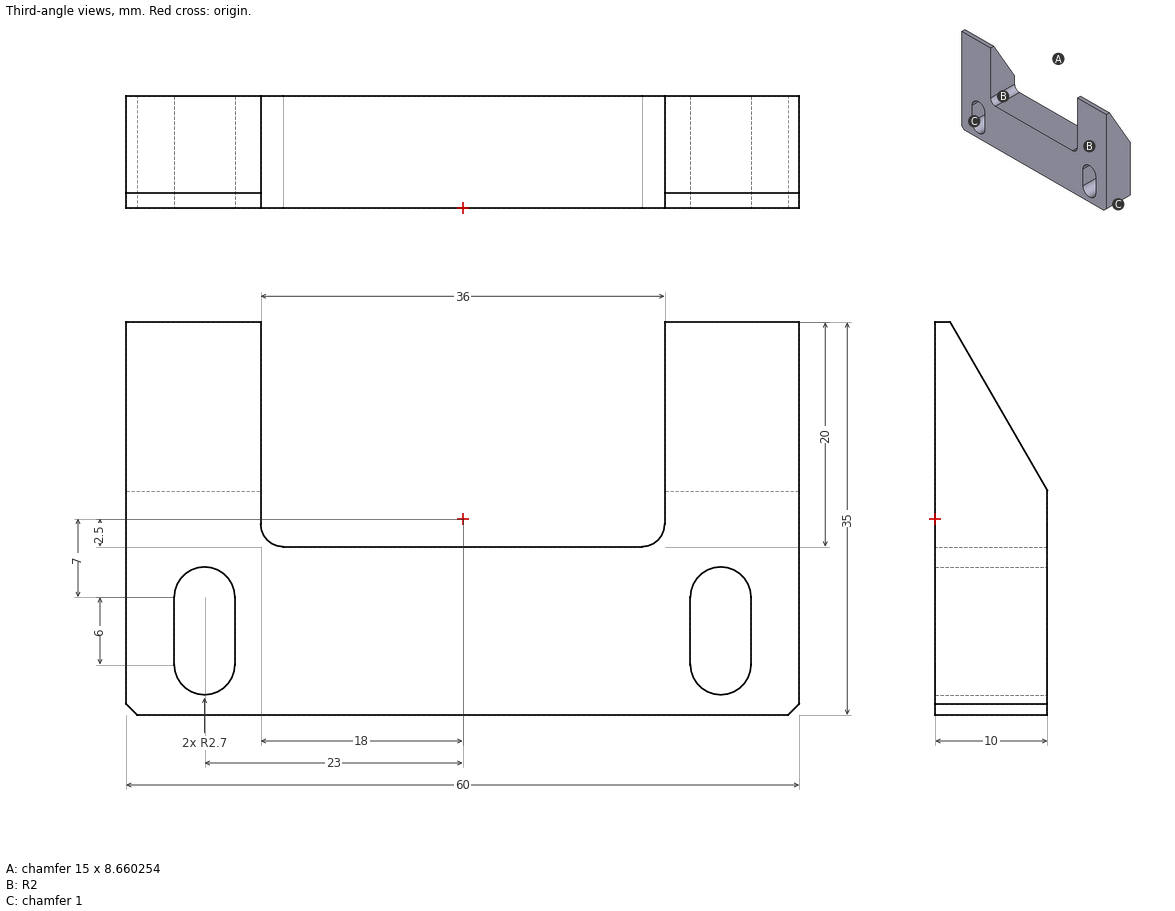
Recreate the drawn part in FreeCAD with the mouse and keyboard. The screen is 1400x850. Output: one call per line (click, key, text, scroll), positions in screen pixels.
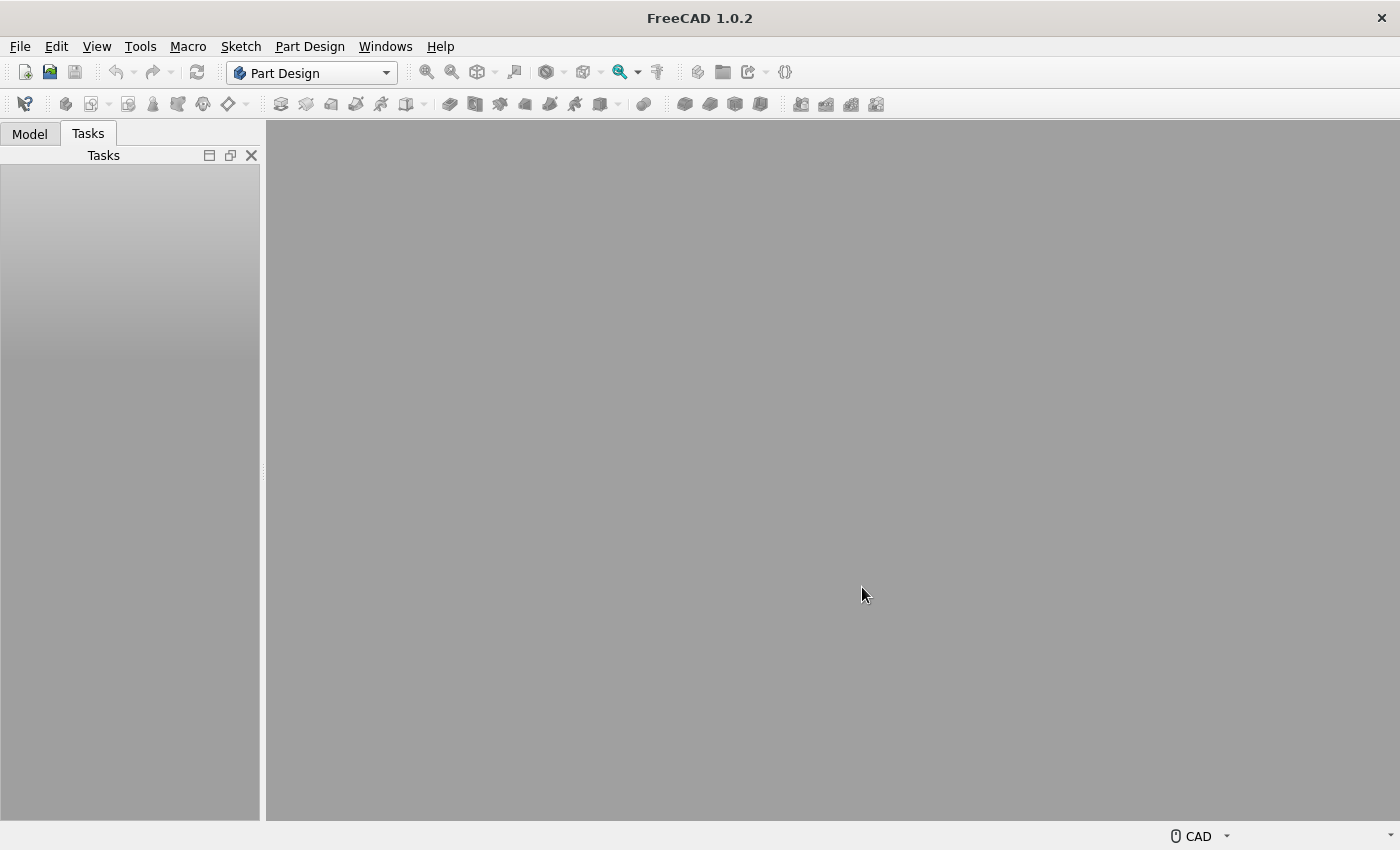
click(25, 72)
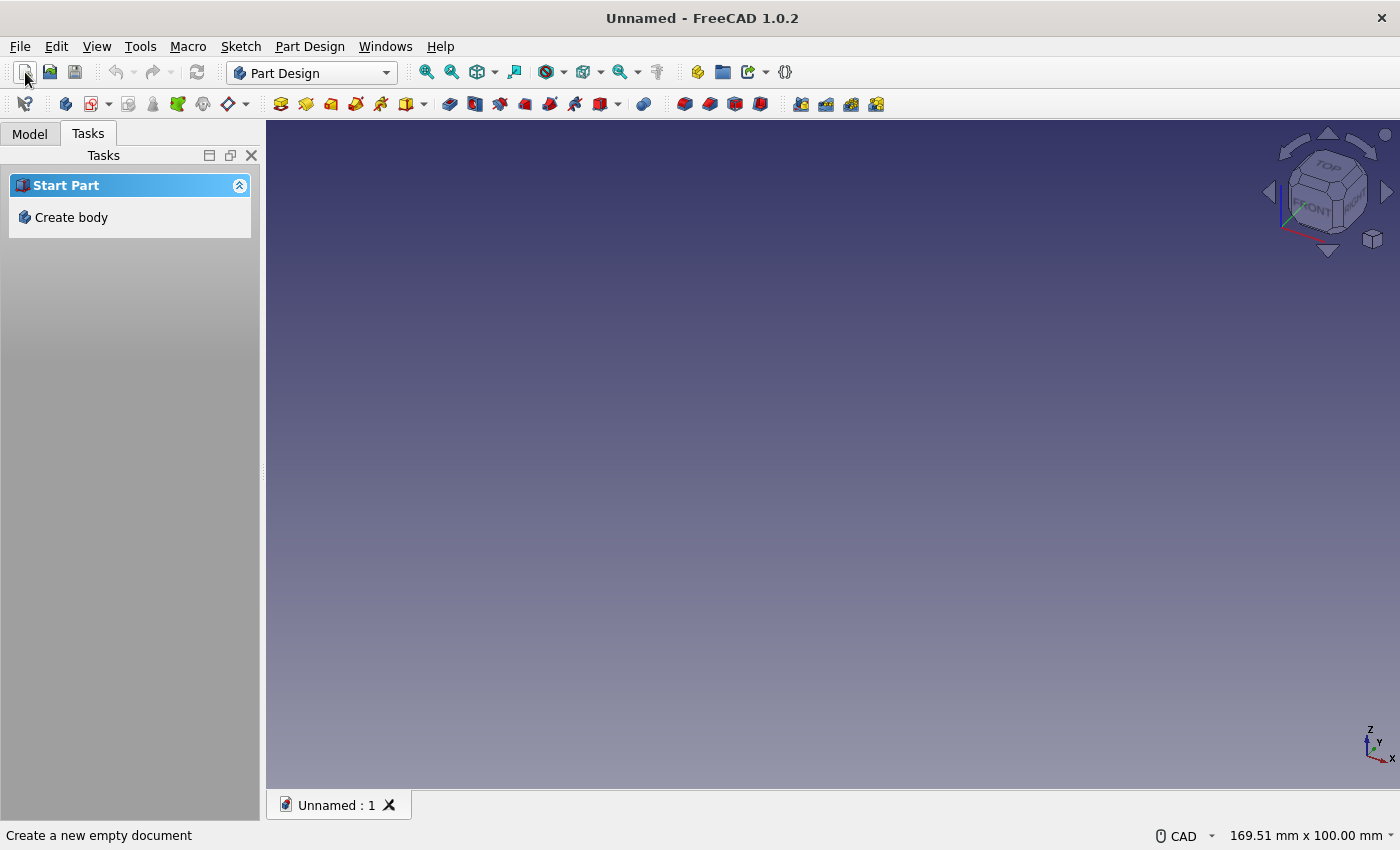
click(90, 104)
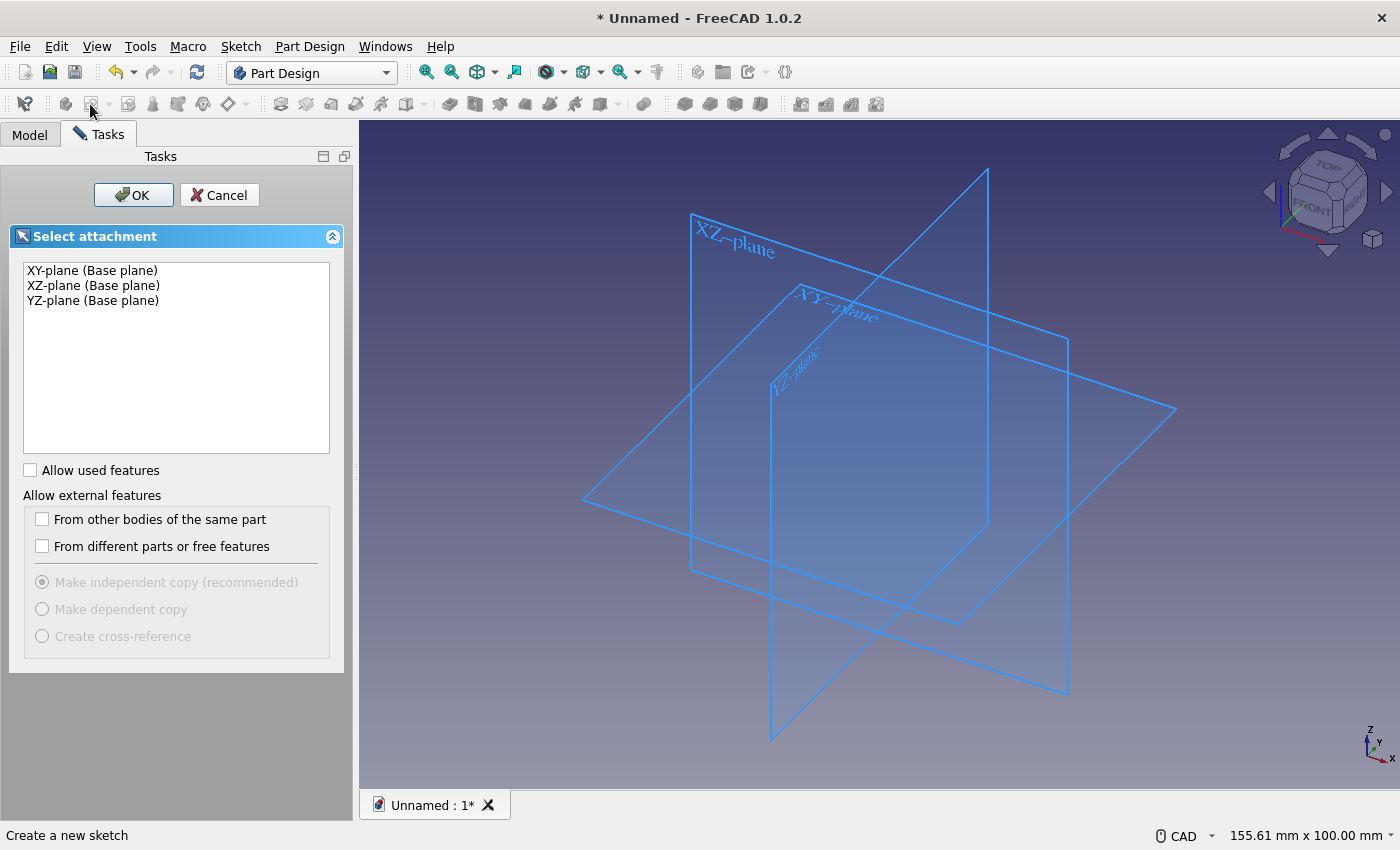
click(84, 286)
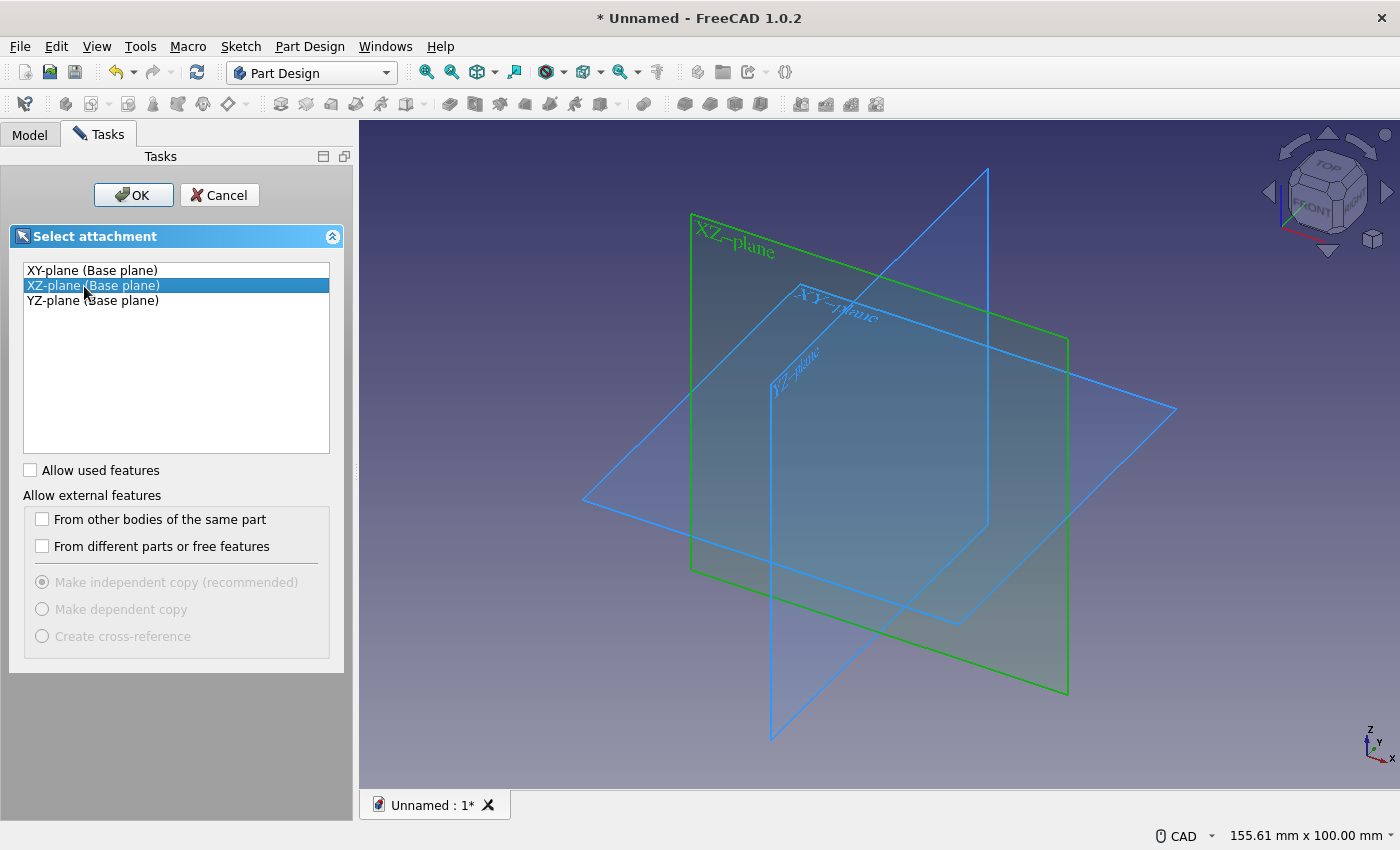
click(134, 195)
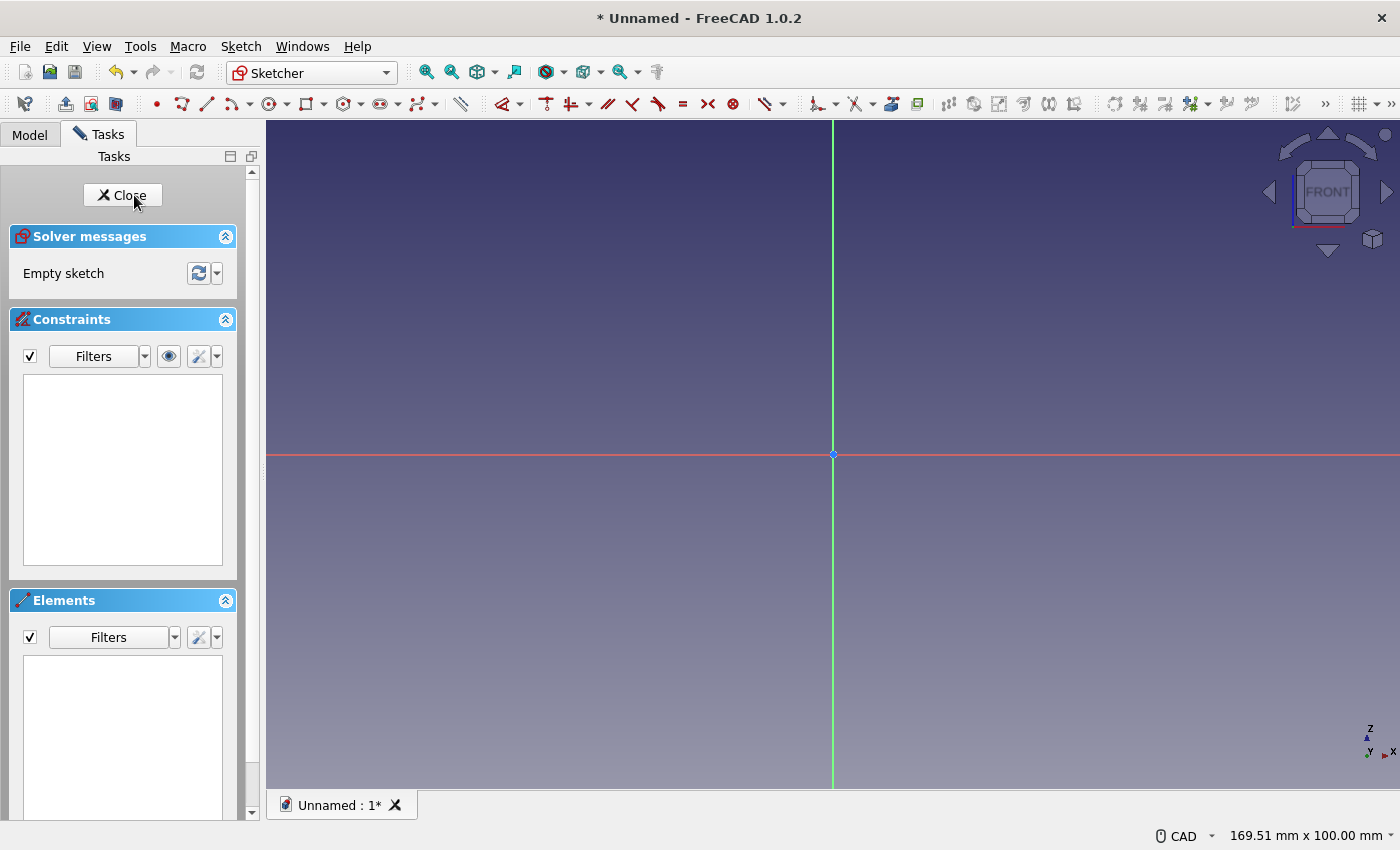
scroll(916, 454, up, 3)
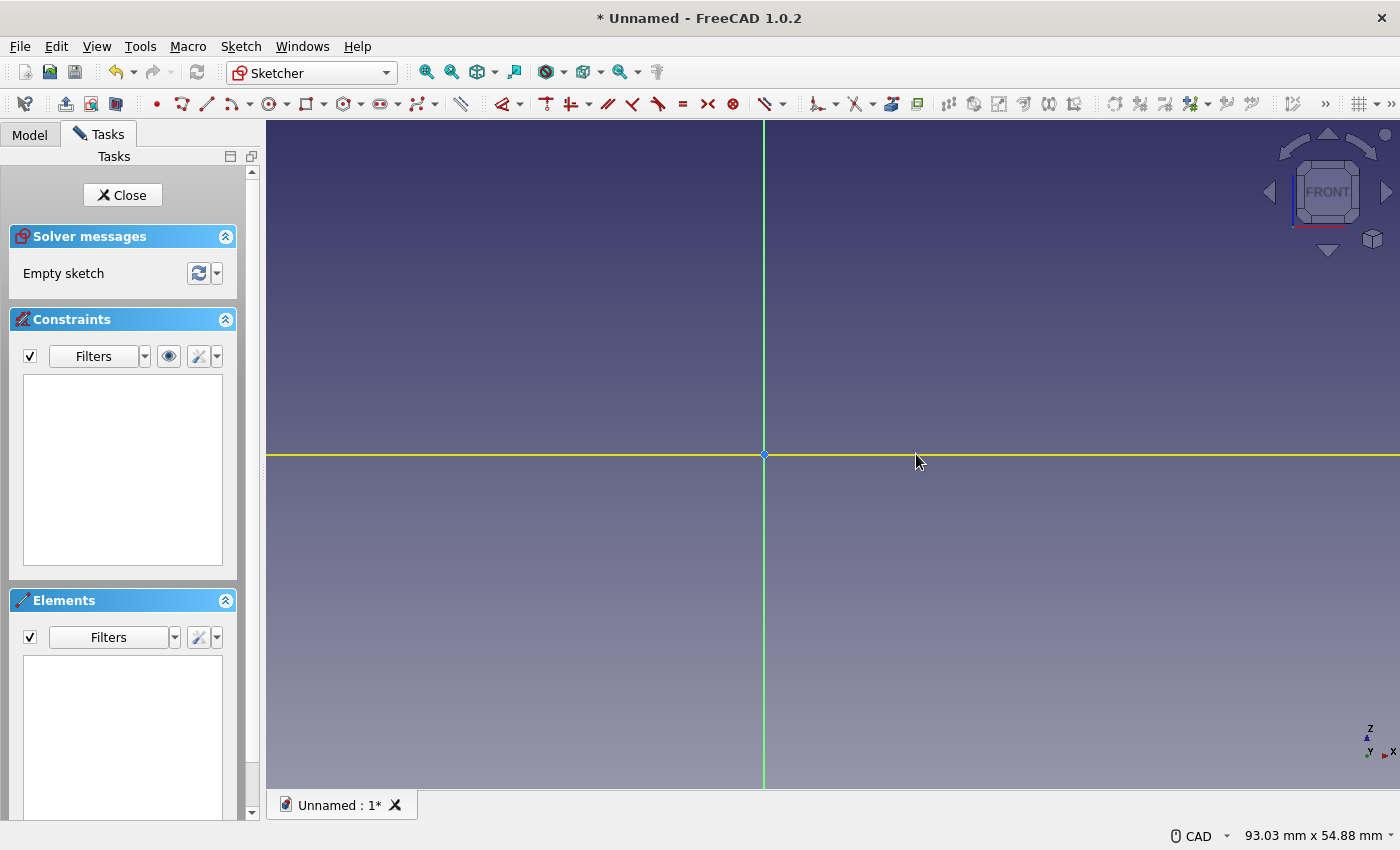
key(g)
key(v)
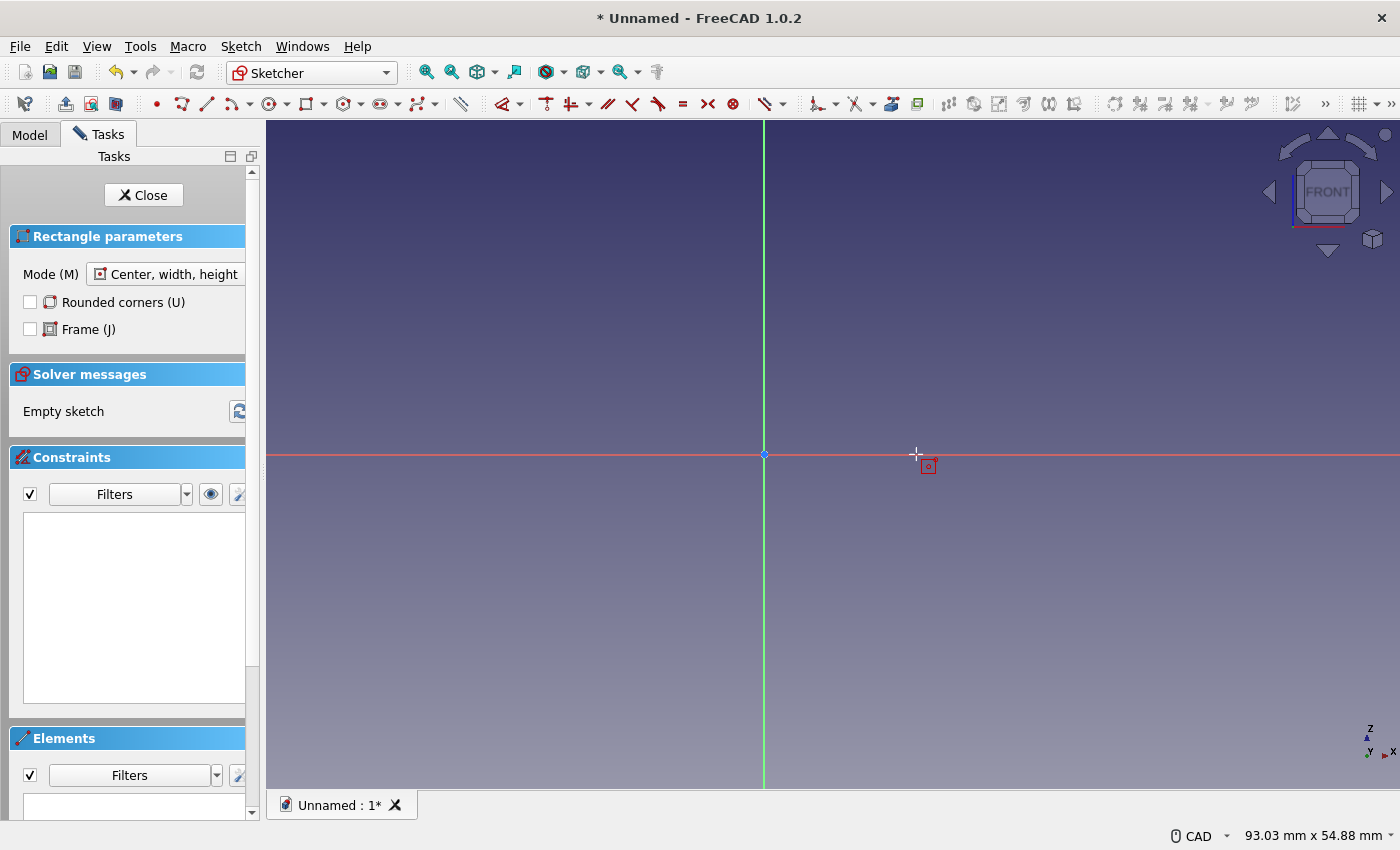
click(764, 454)
move(1130, 241)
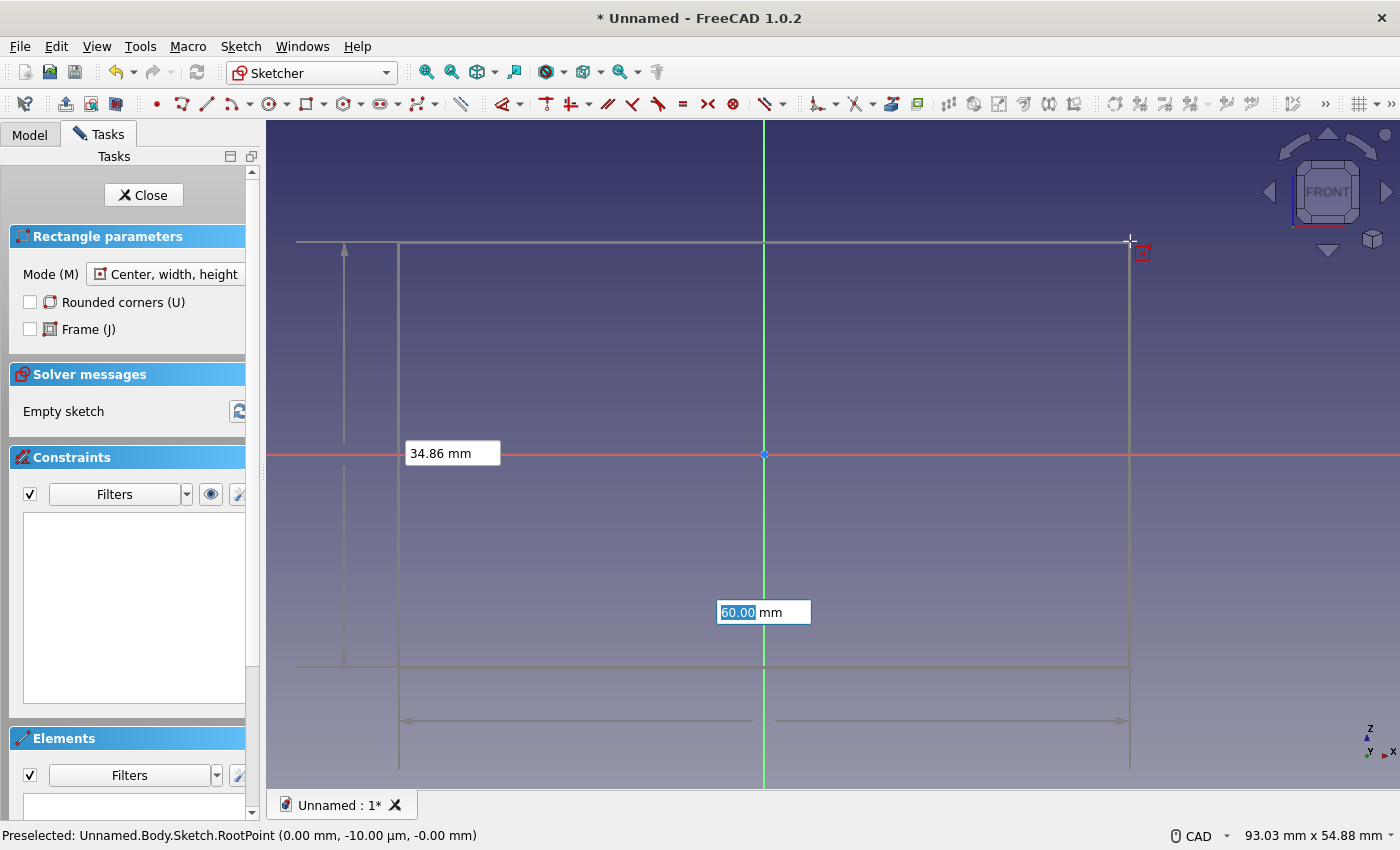
text(60)
key(Tab)
text(35)
key(Return)
key(Escape)